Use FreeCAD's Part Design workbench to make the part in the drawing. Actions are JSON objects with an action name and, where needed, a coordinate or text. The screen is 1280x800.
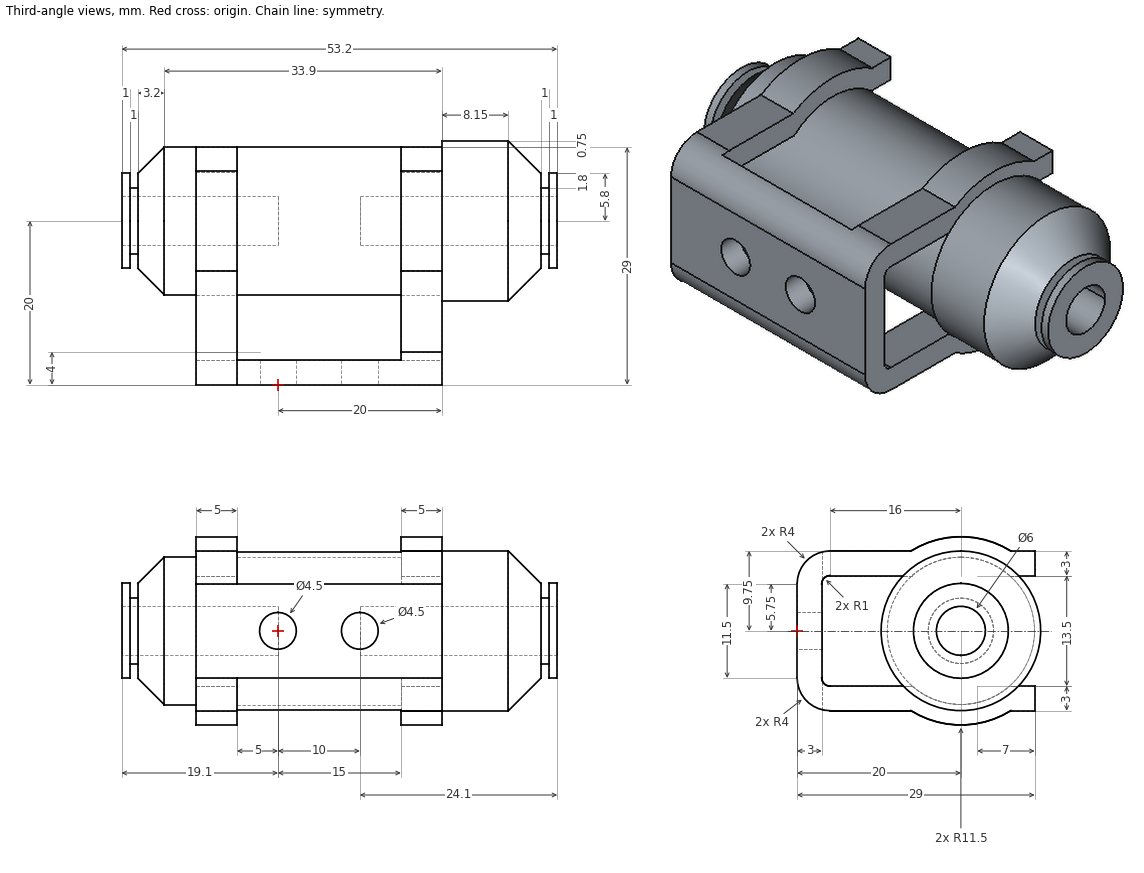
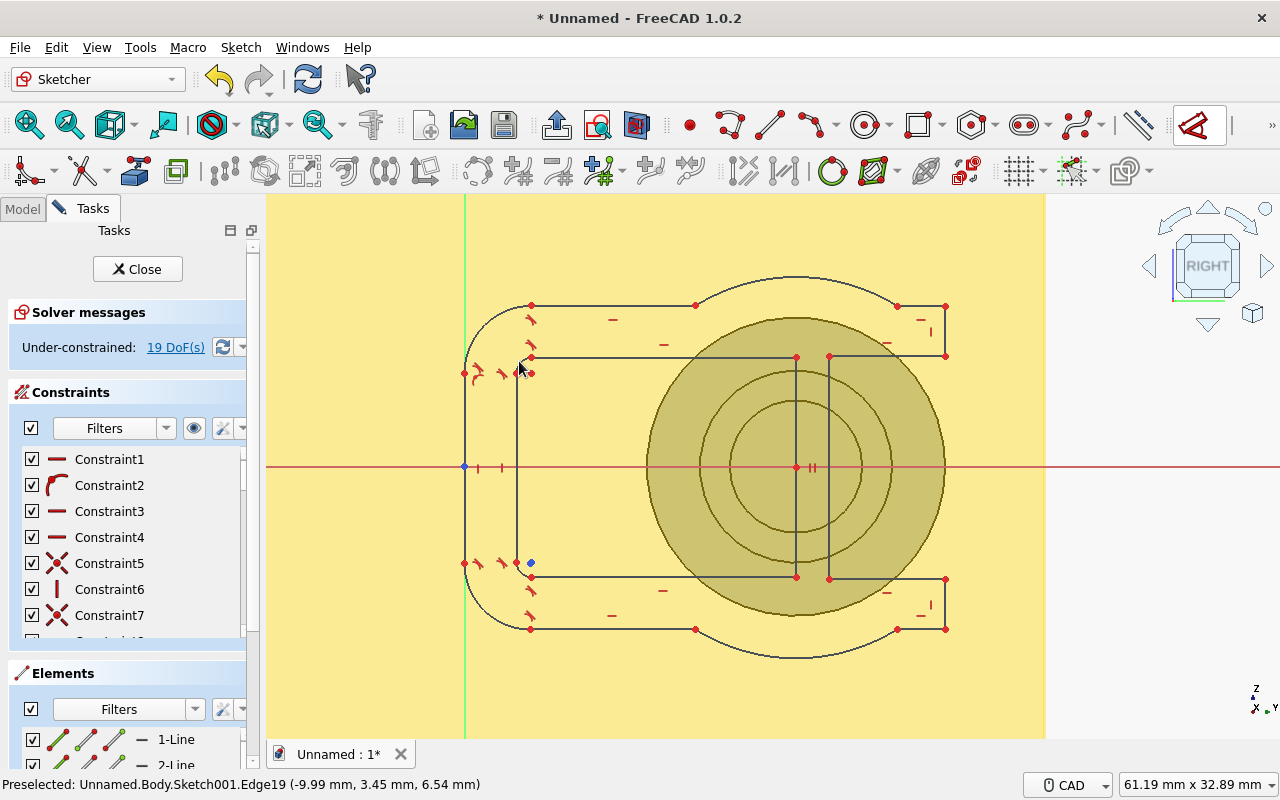
{"action": "left_click", "coordinate": [500, 622]}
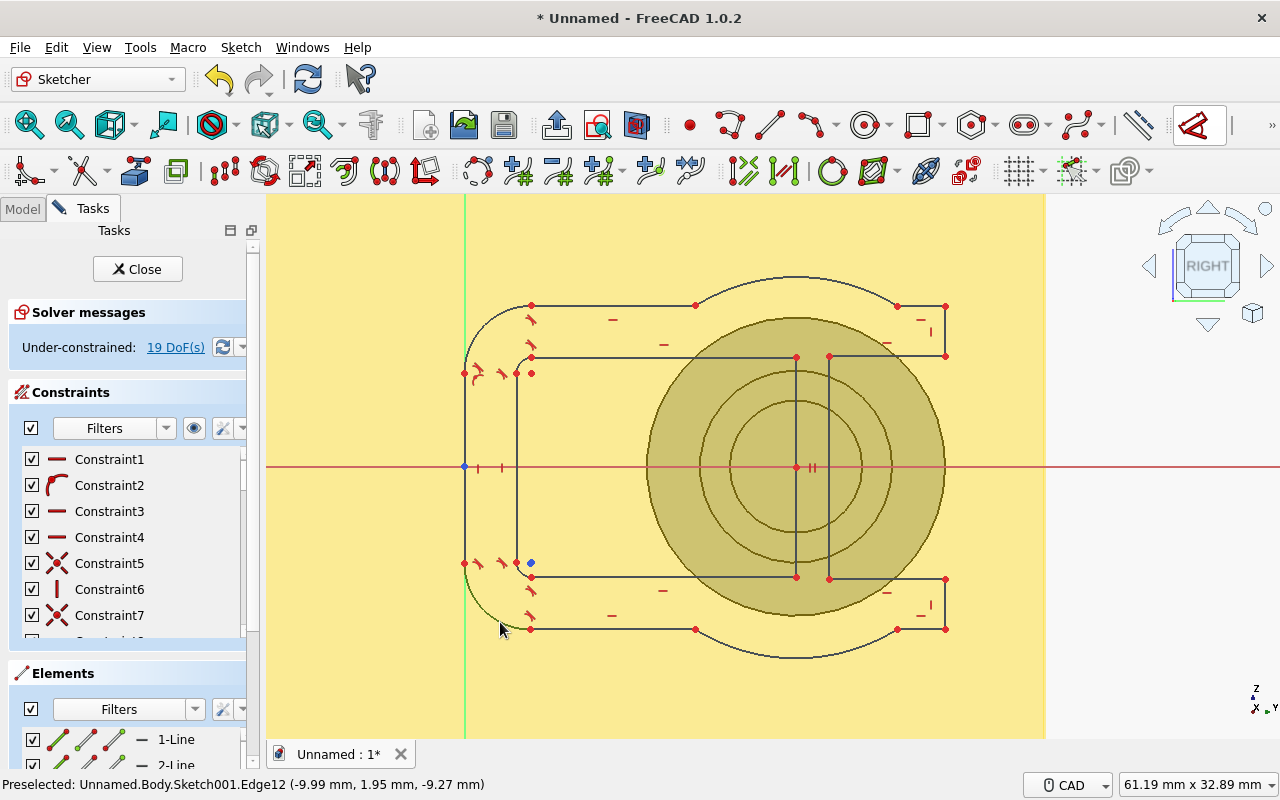
{"action": "left_click", "coordinate": [521, 573]}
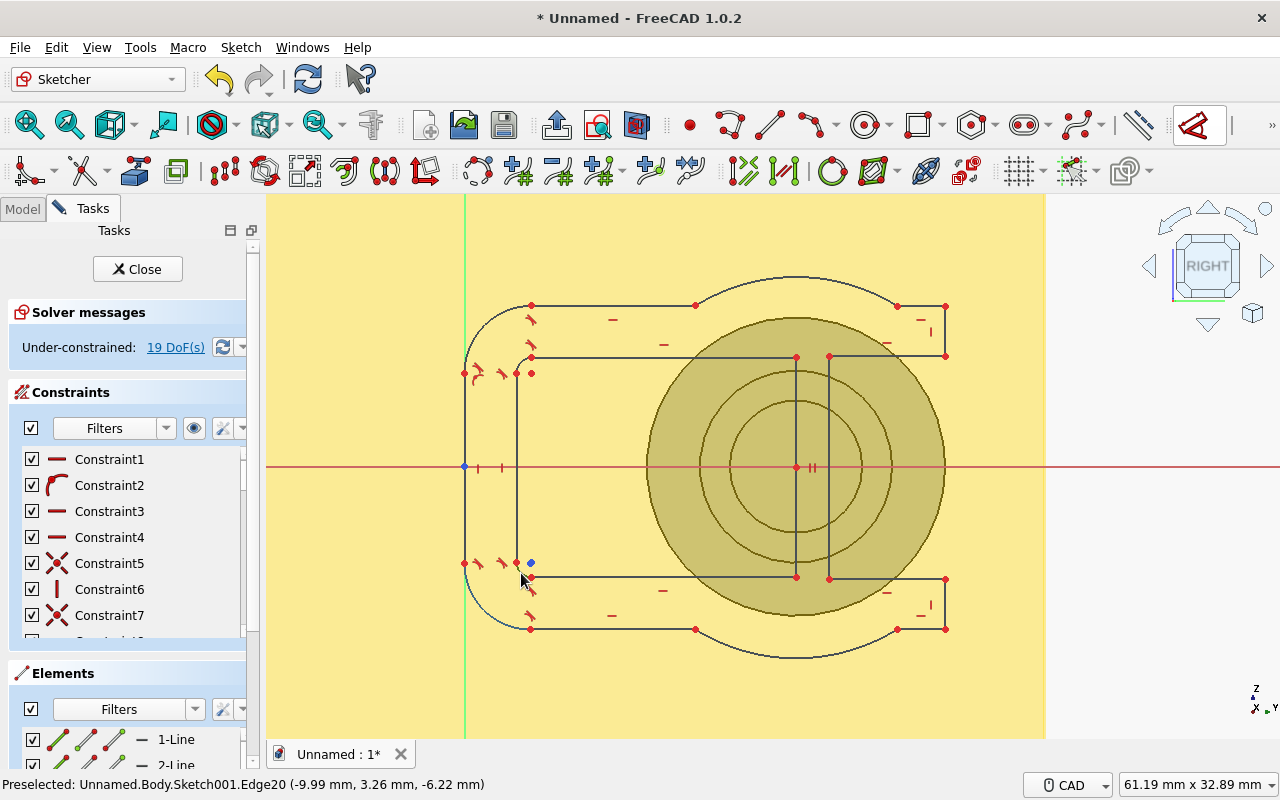
{"action": "key", "text": "c"}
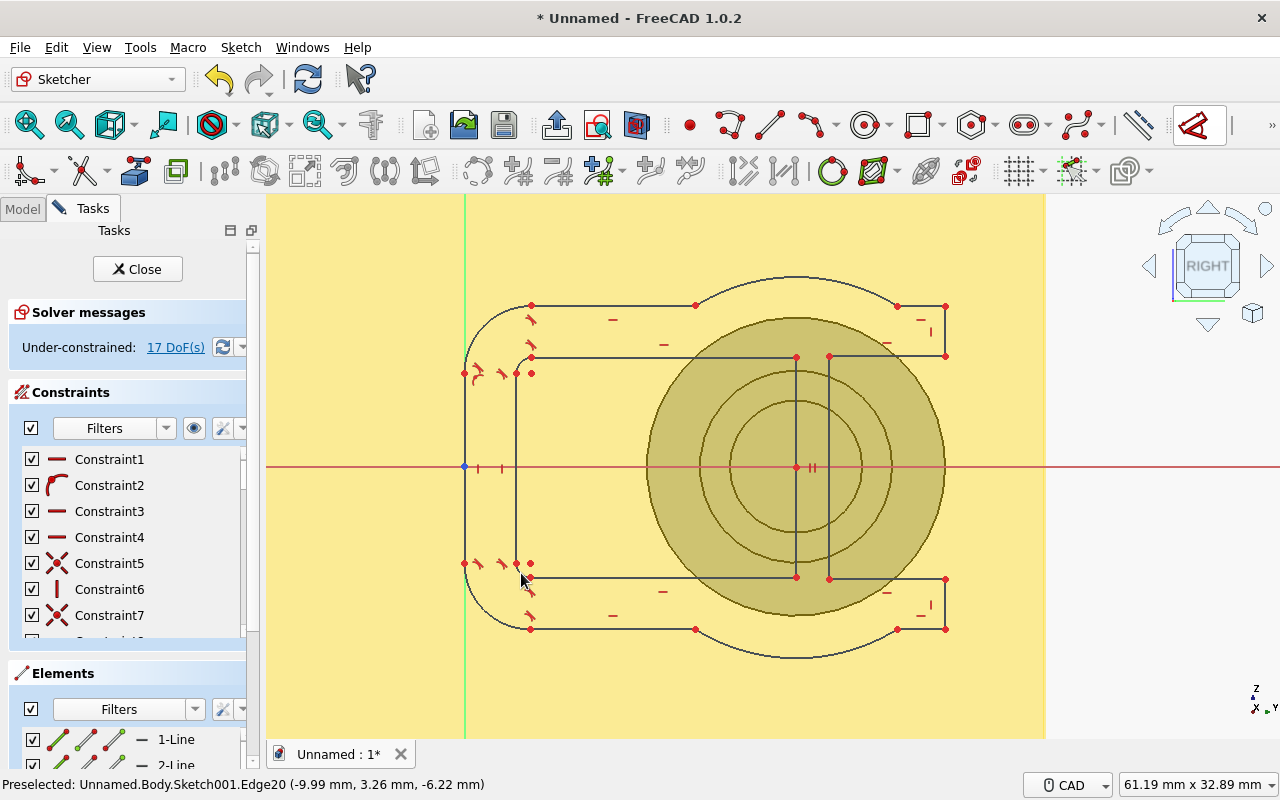
{"action": "left_click", "coordinate": [501, 313]}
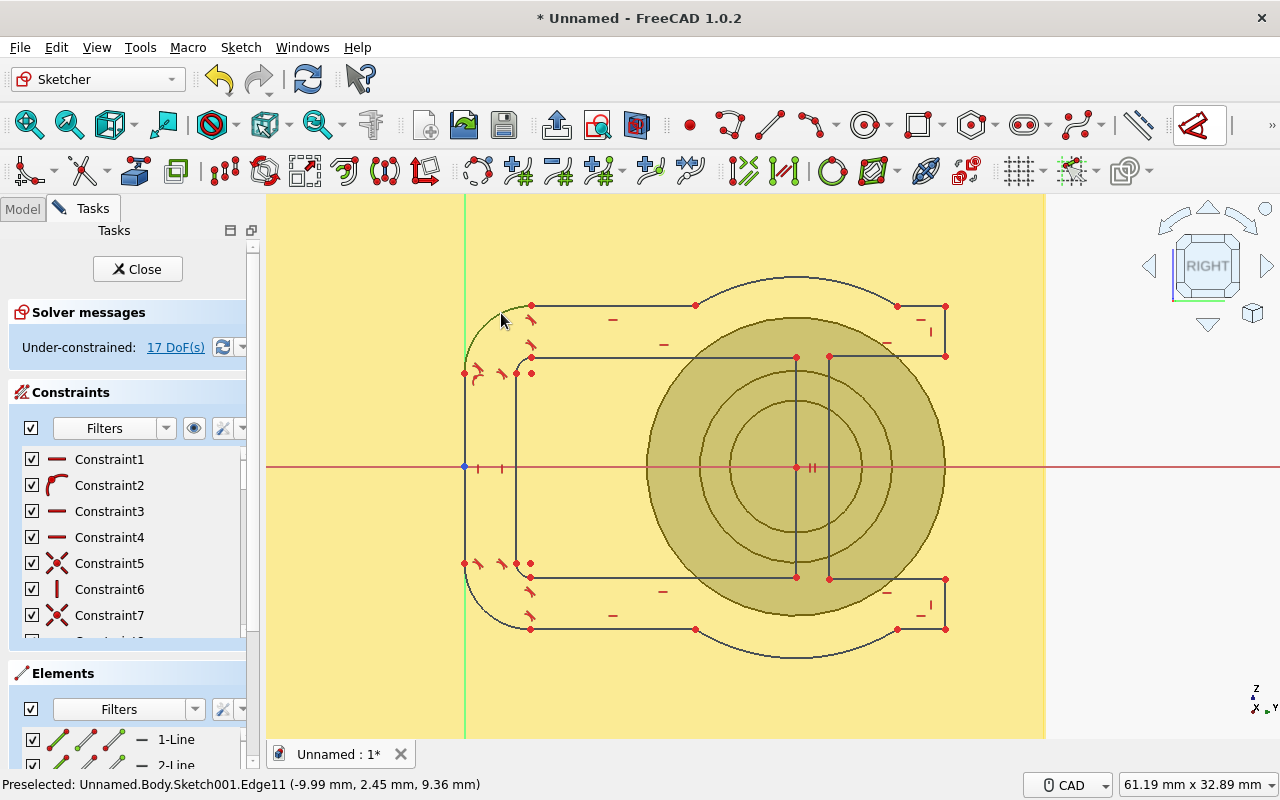
{"action": "left_click", "coordinate": [501, 622]}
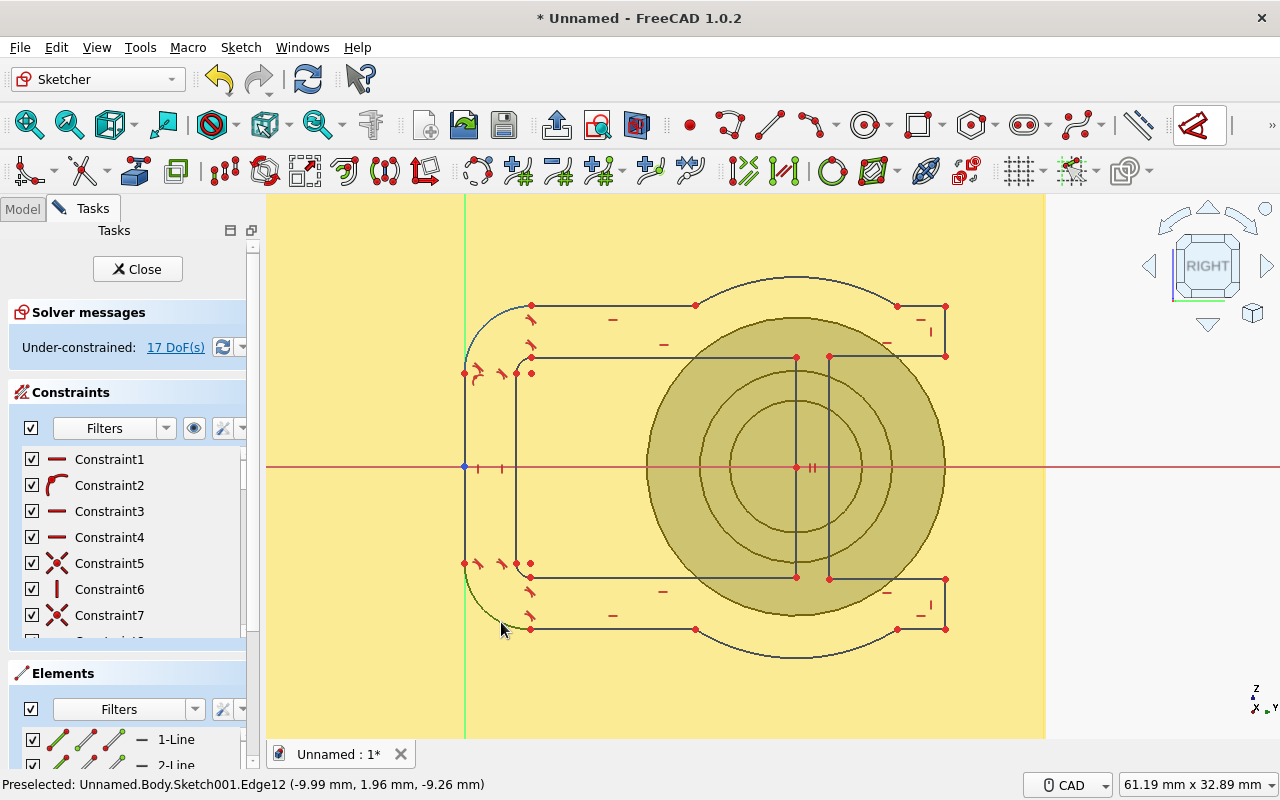
{"action": "key", "text": "e"}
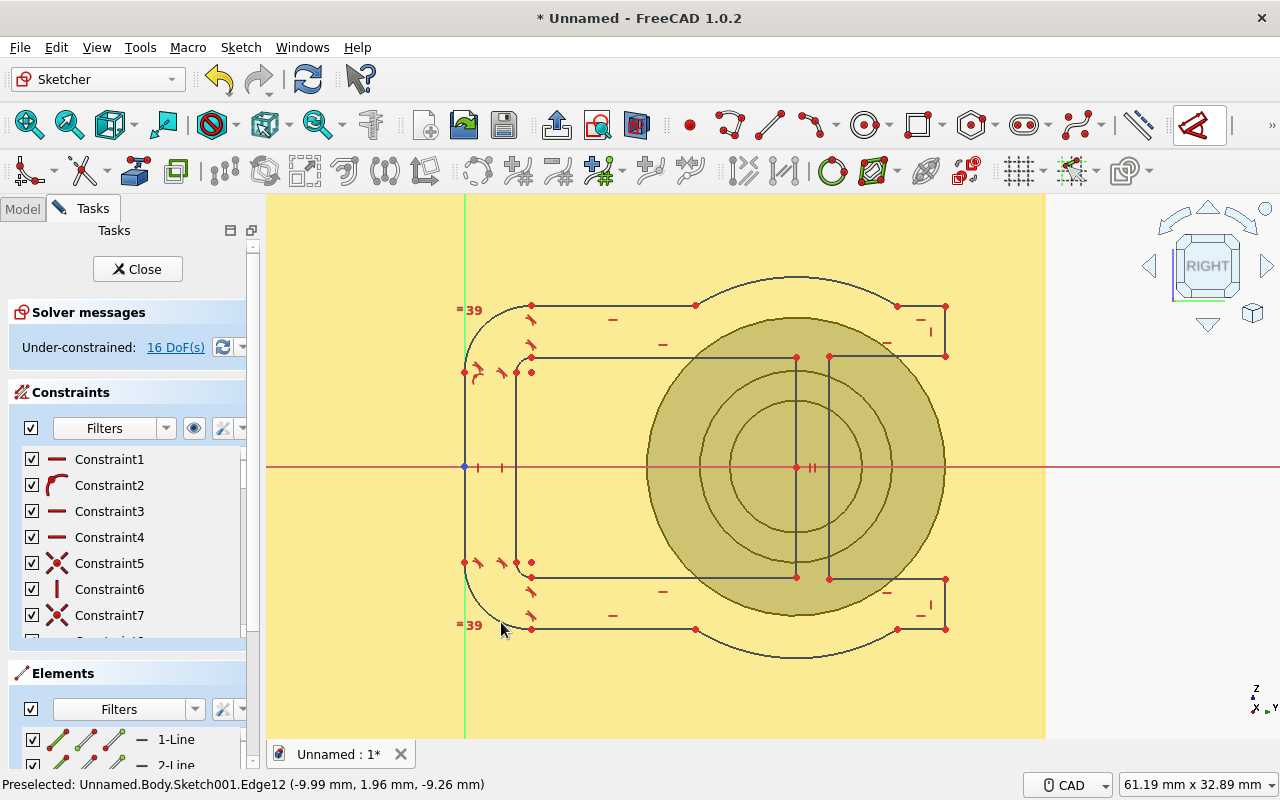
{"action": "left_click", "coordinate": [754, 654]}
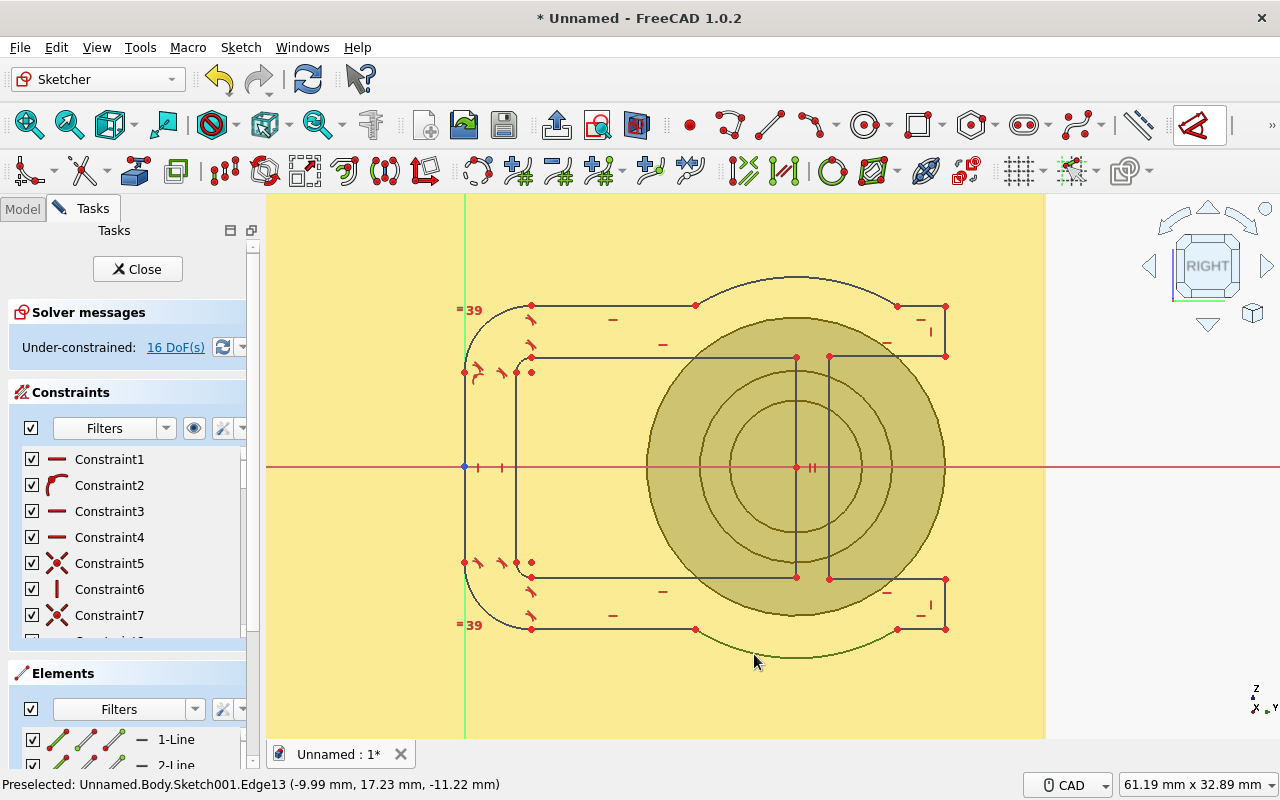
{"action": "left_click", "coordinate": [839, 282]}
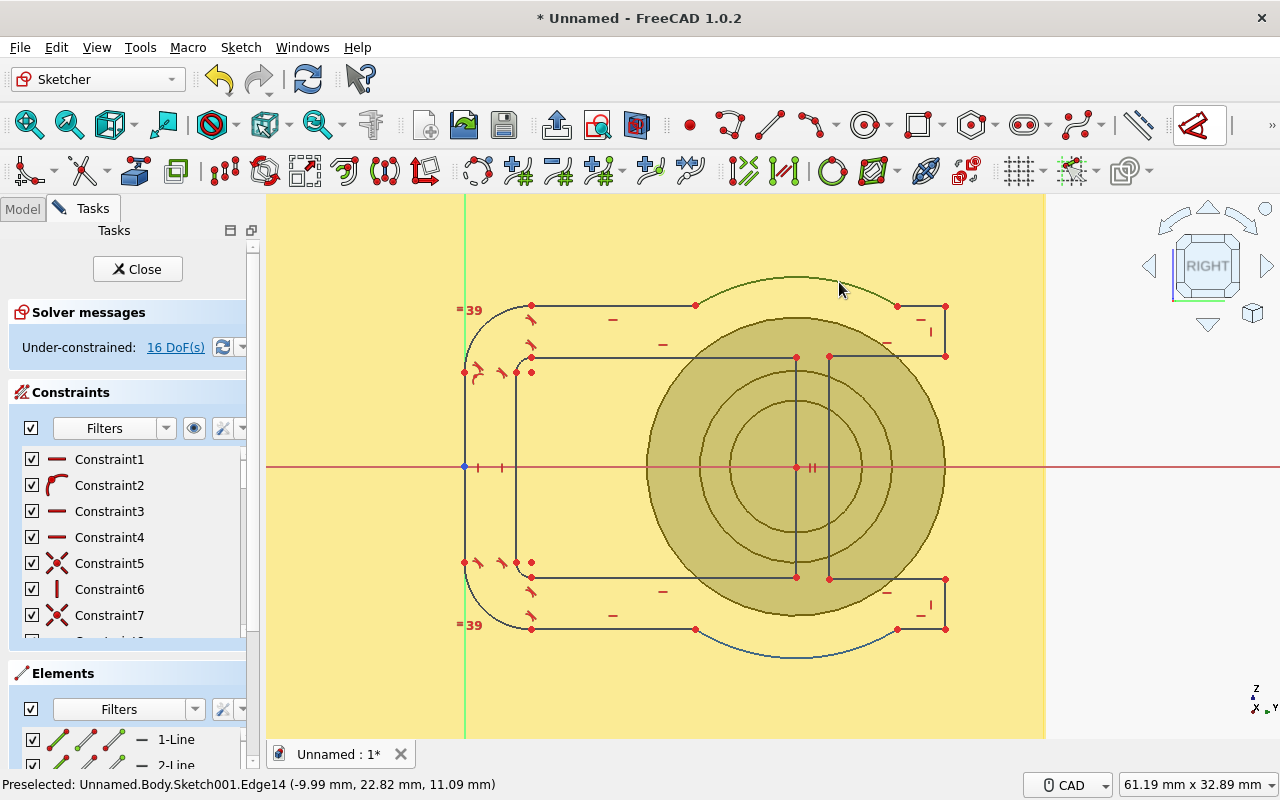
{"action": "key", "text": "e"}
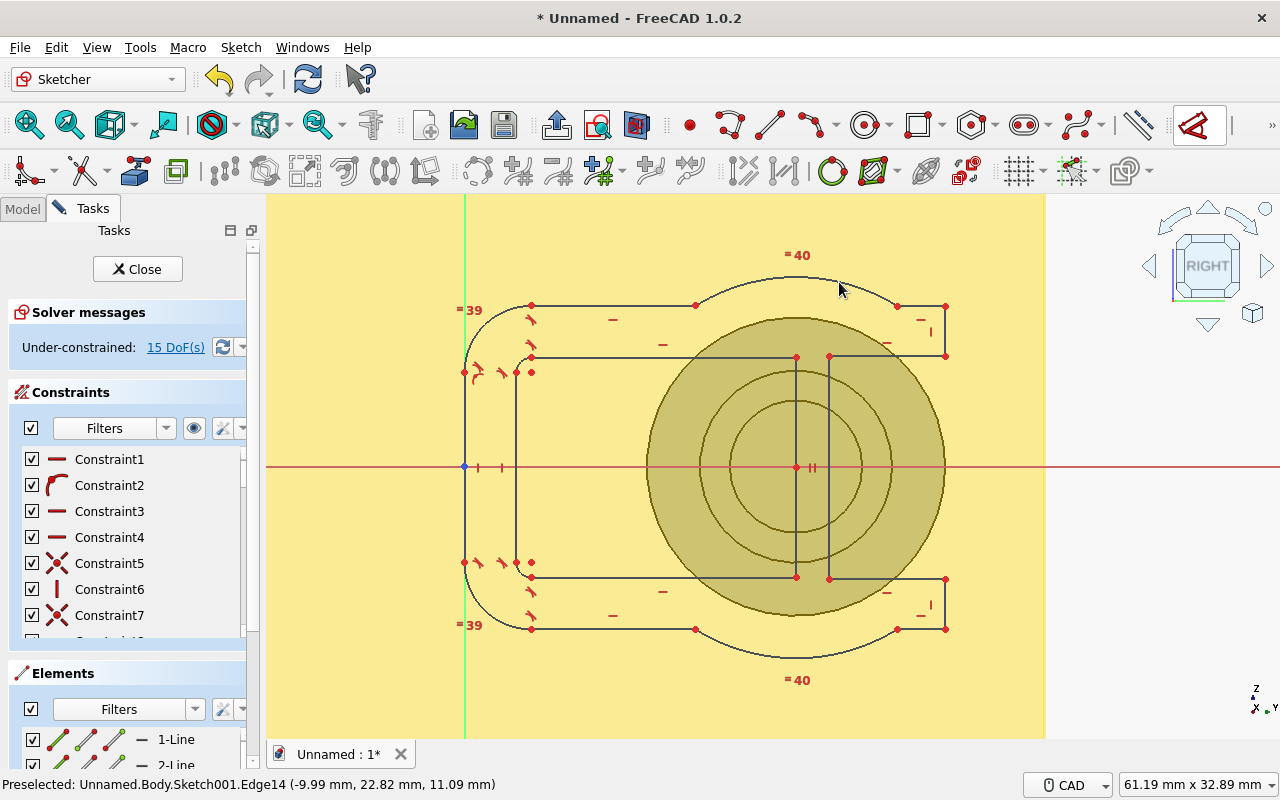
{"action": "left_click", "coordinate": [796, 468]}